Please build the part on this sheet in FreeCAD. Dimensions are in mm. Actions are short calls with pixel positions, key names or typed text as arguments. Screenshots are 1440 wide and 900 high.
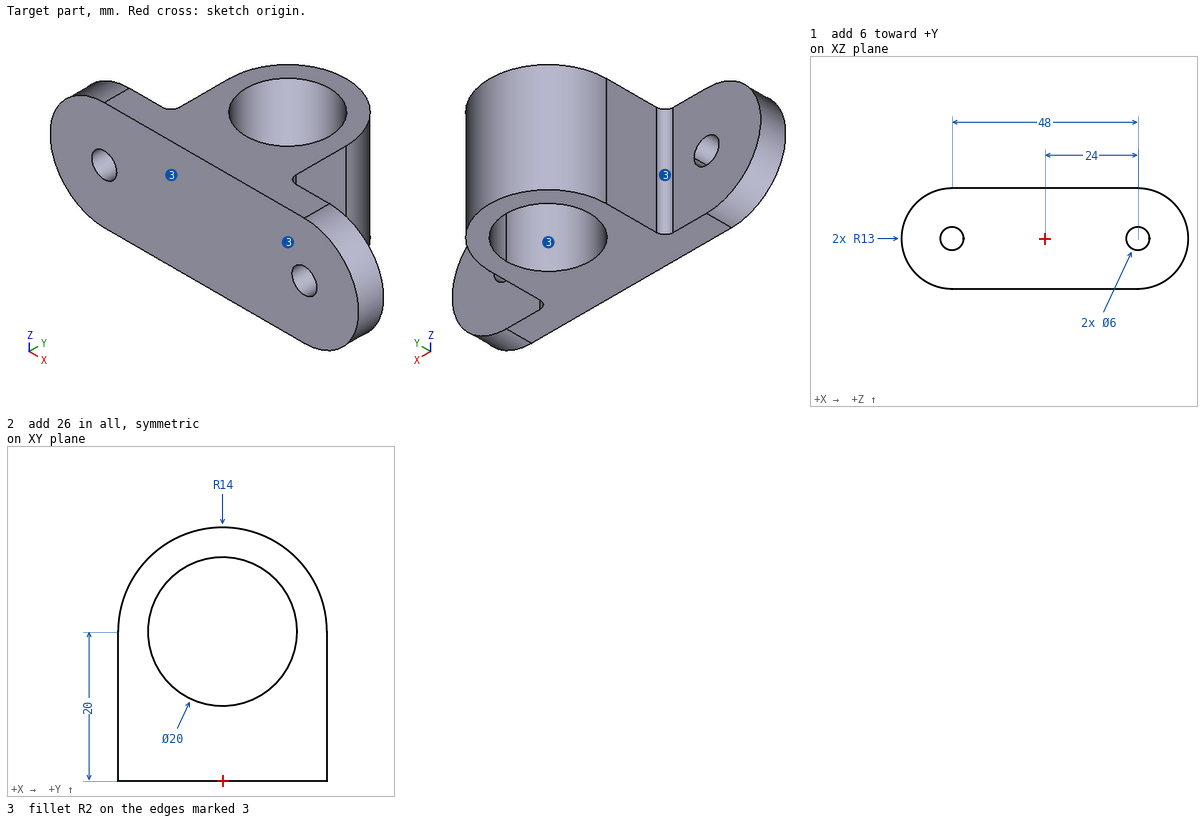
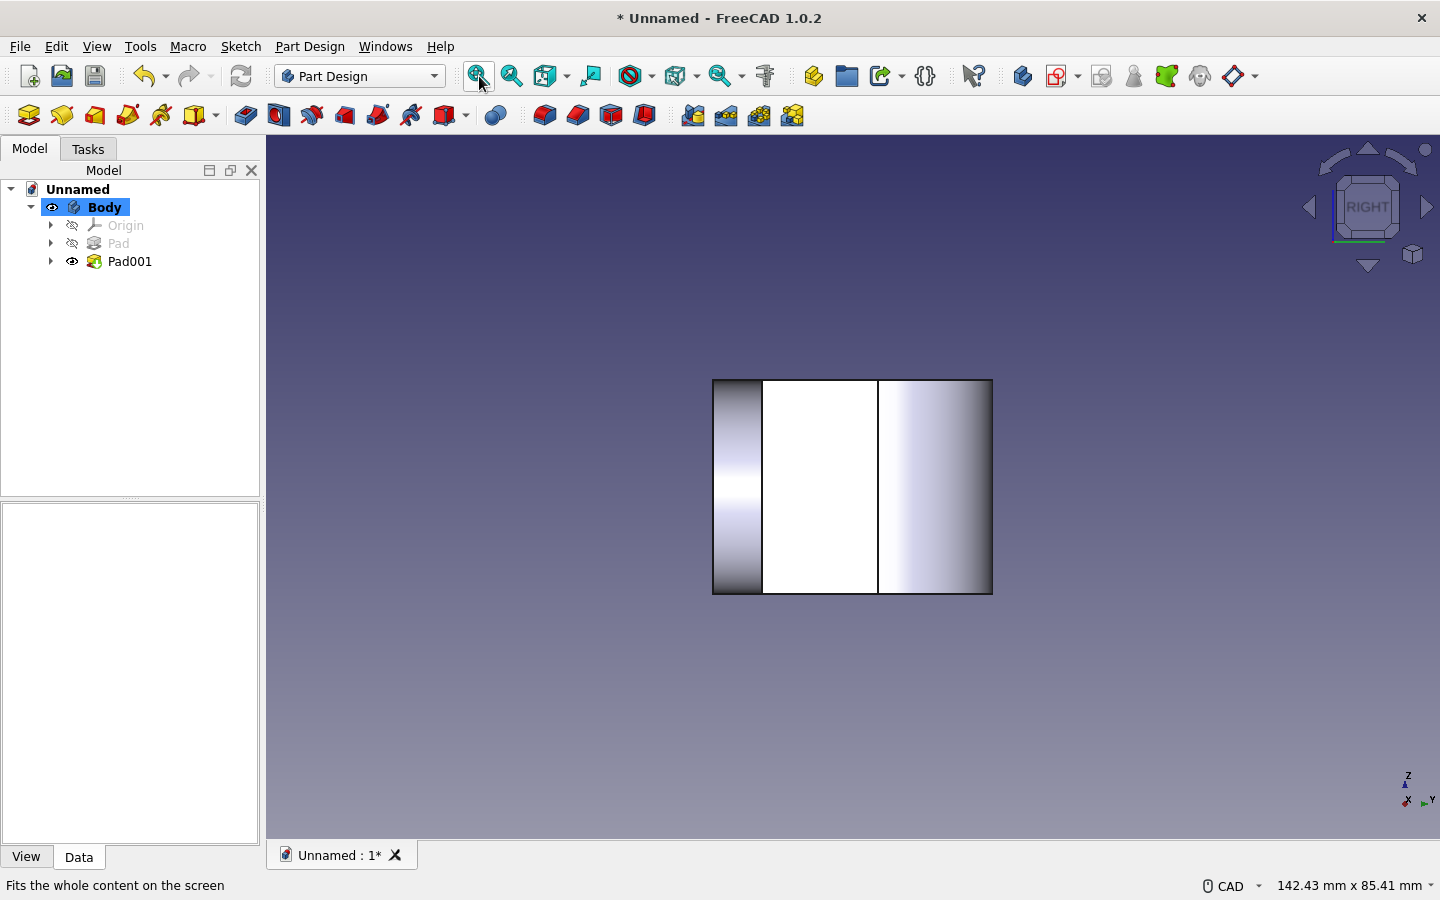
key(5)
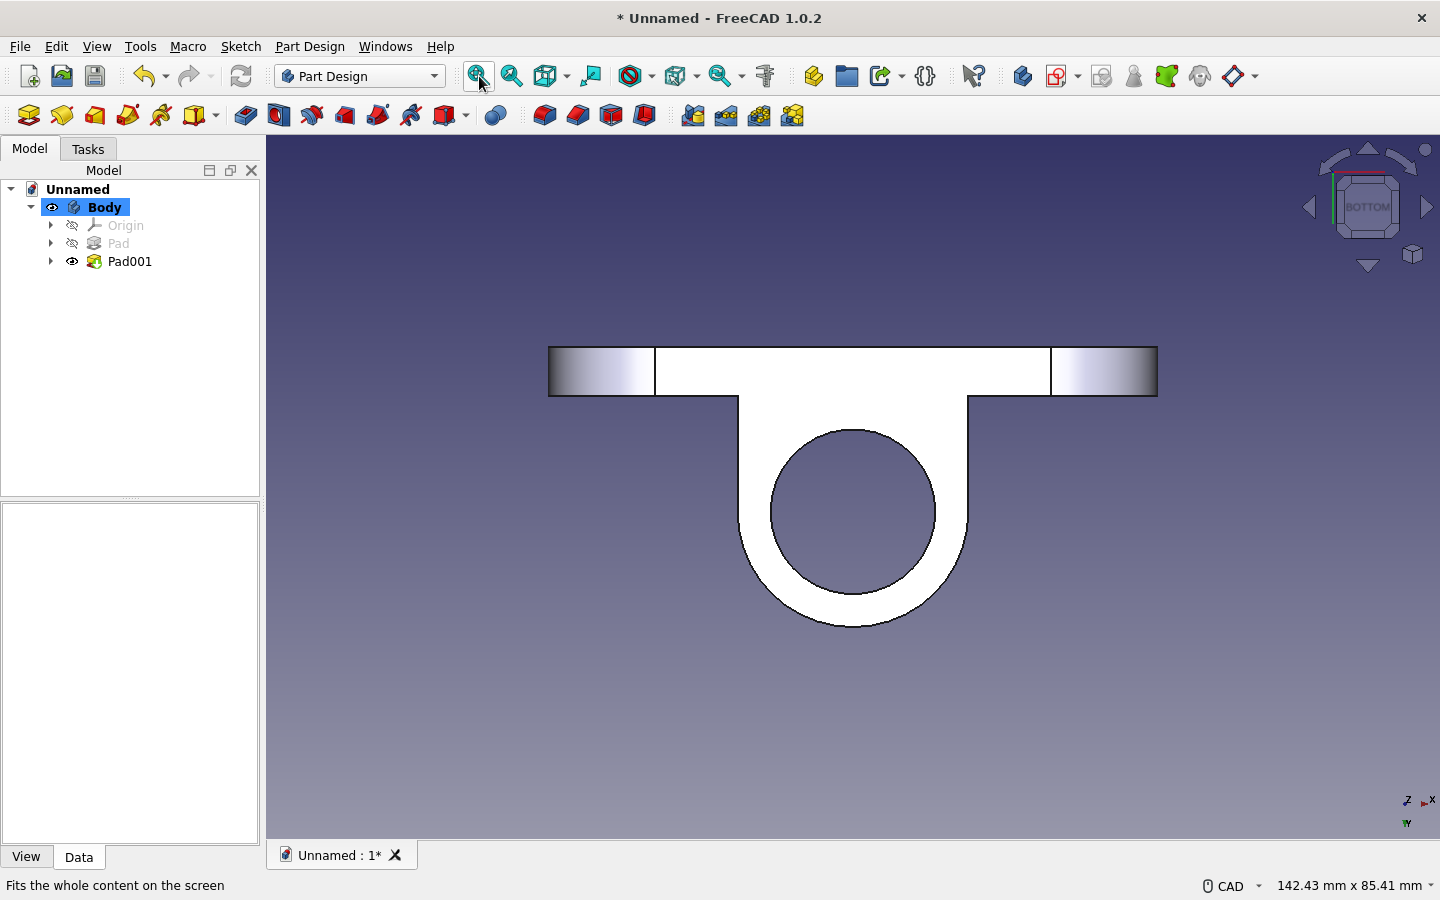
key(4)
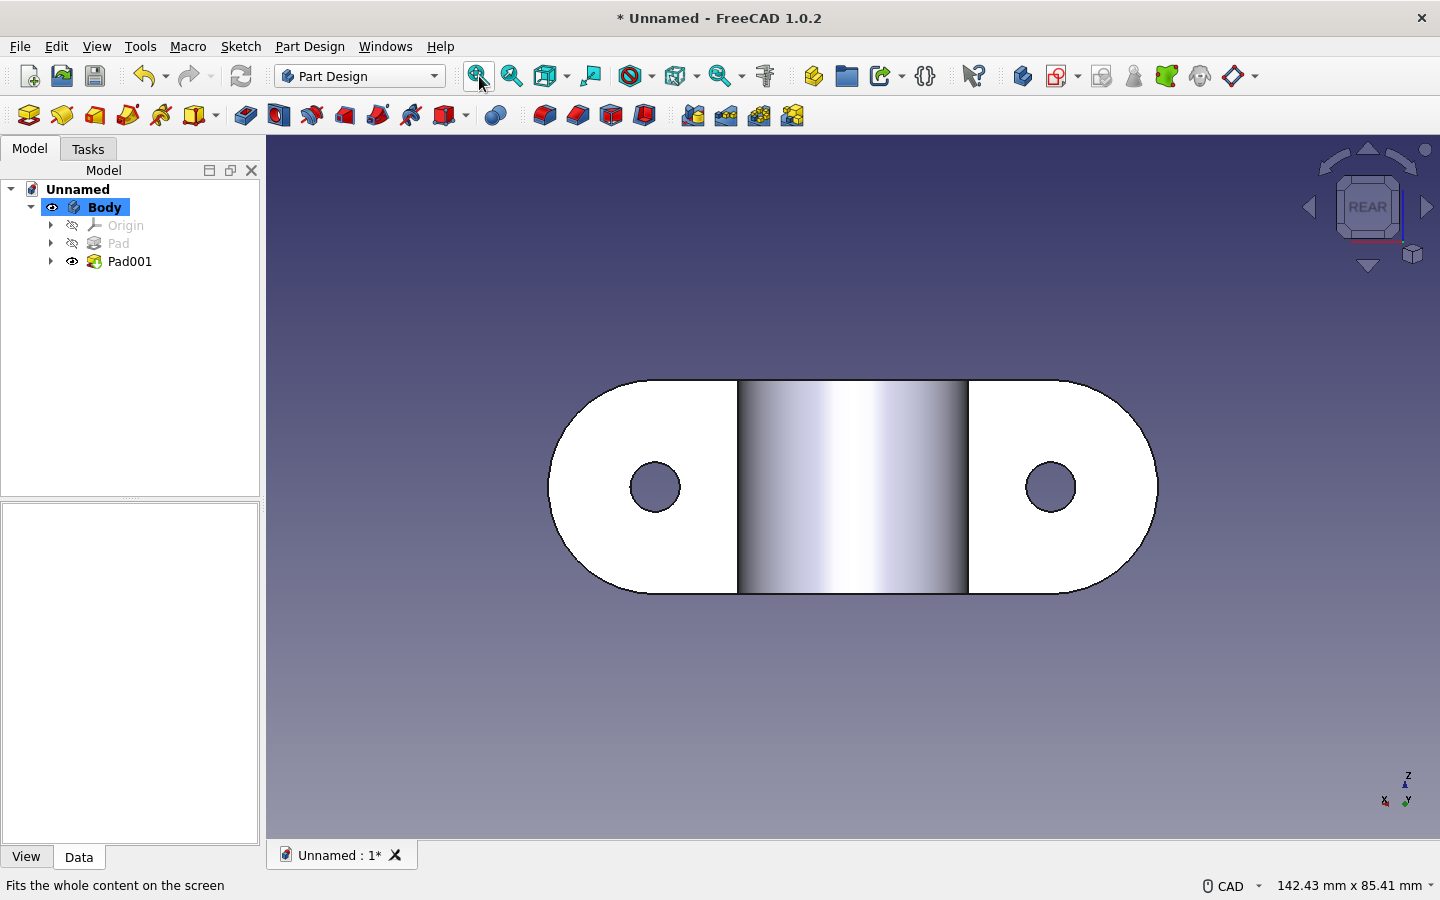
key(6)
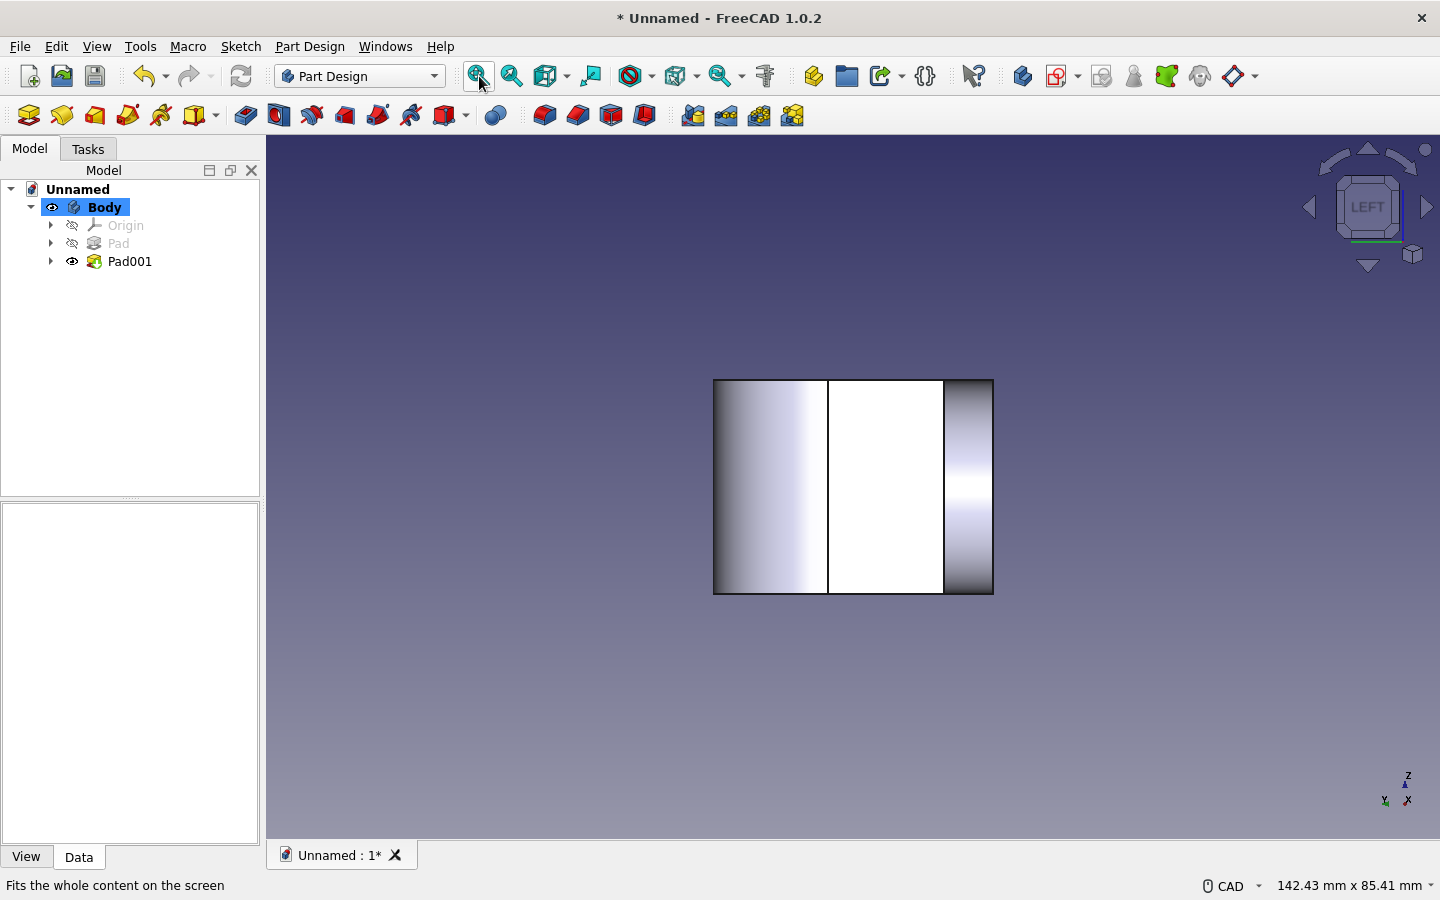
key(v)
key(f)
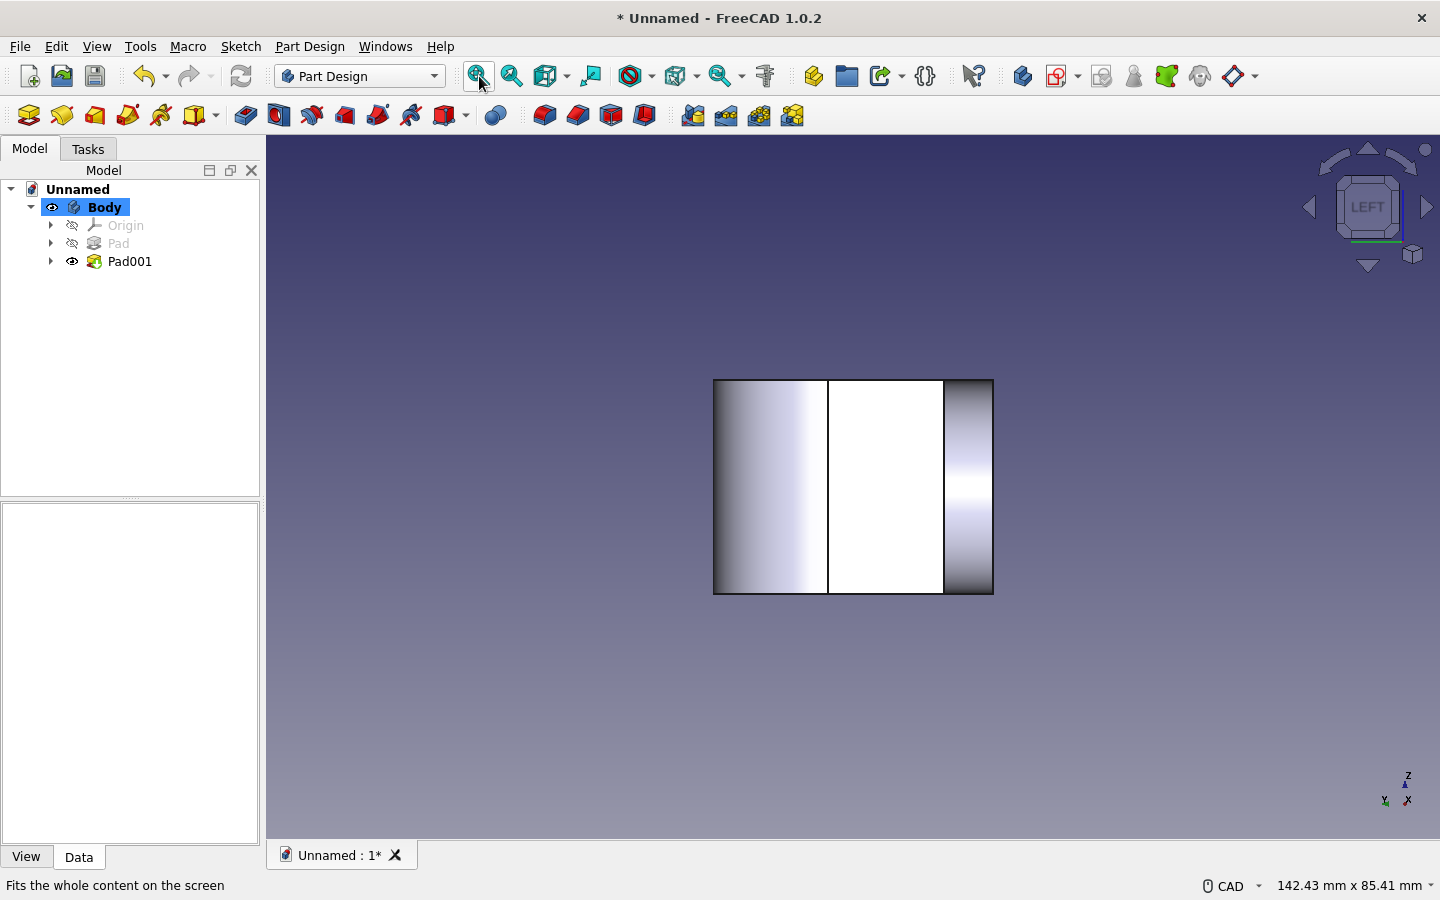
key(v)
key(3)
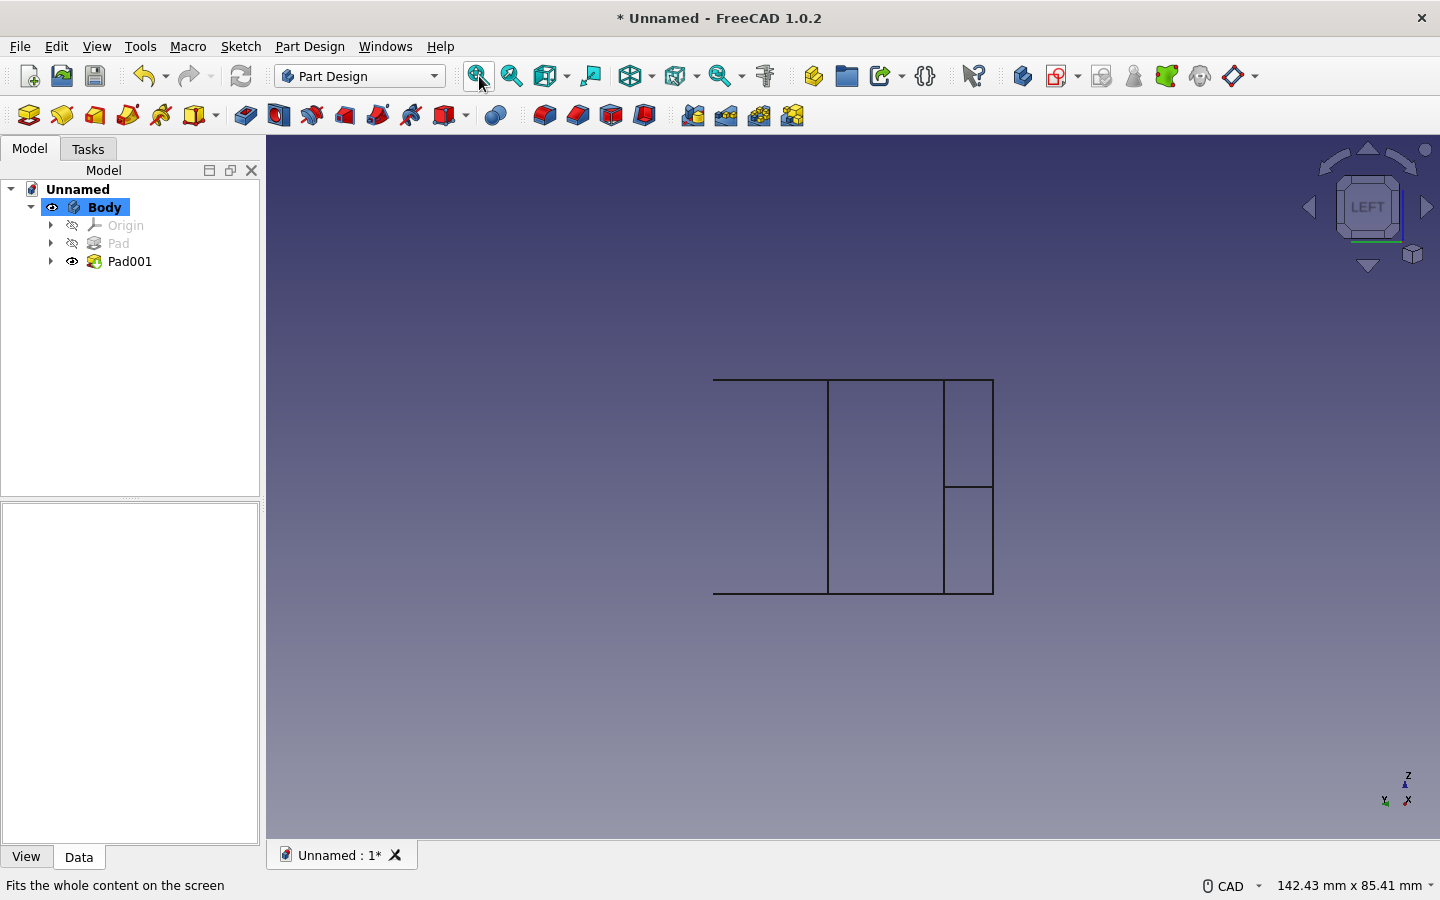
key(0)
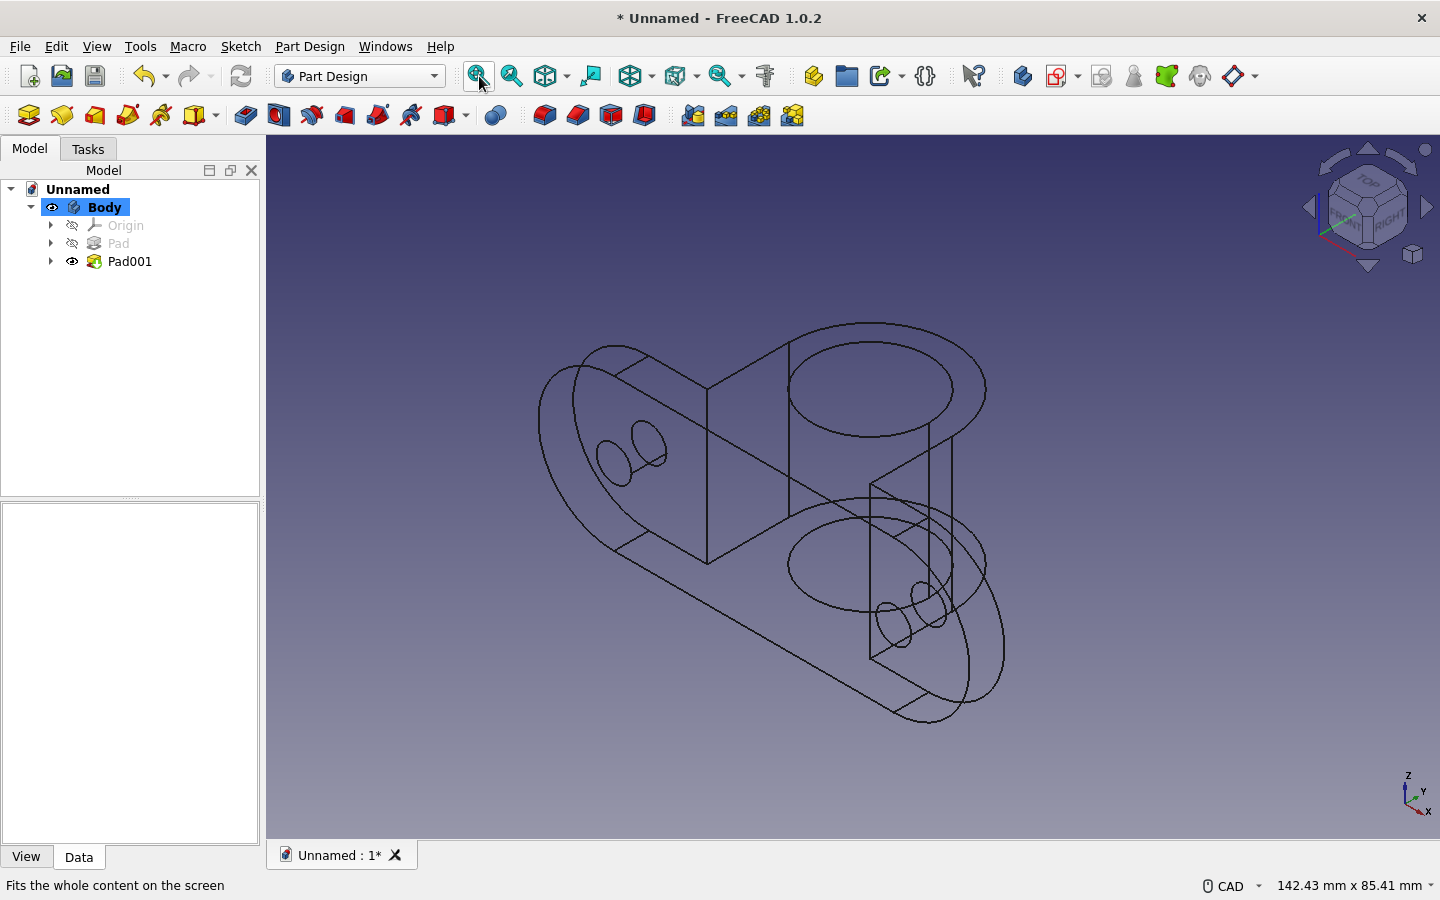
click(707, 476)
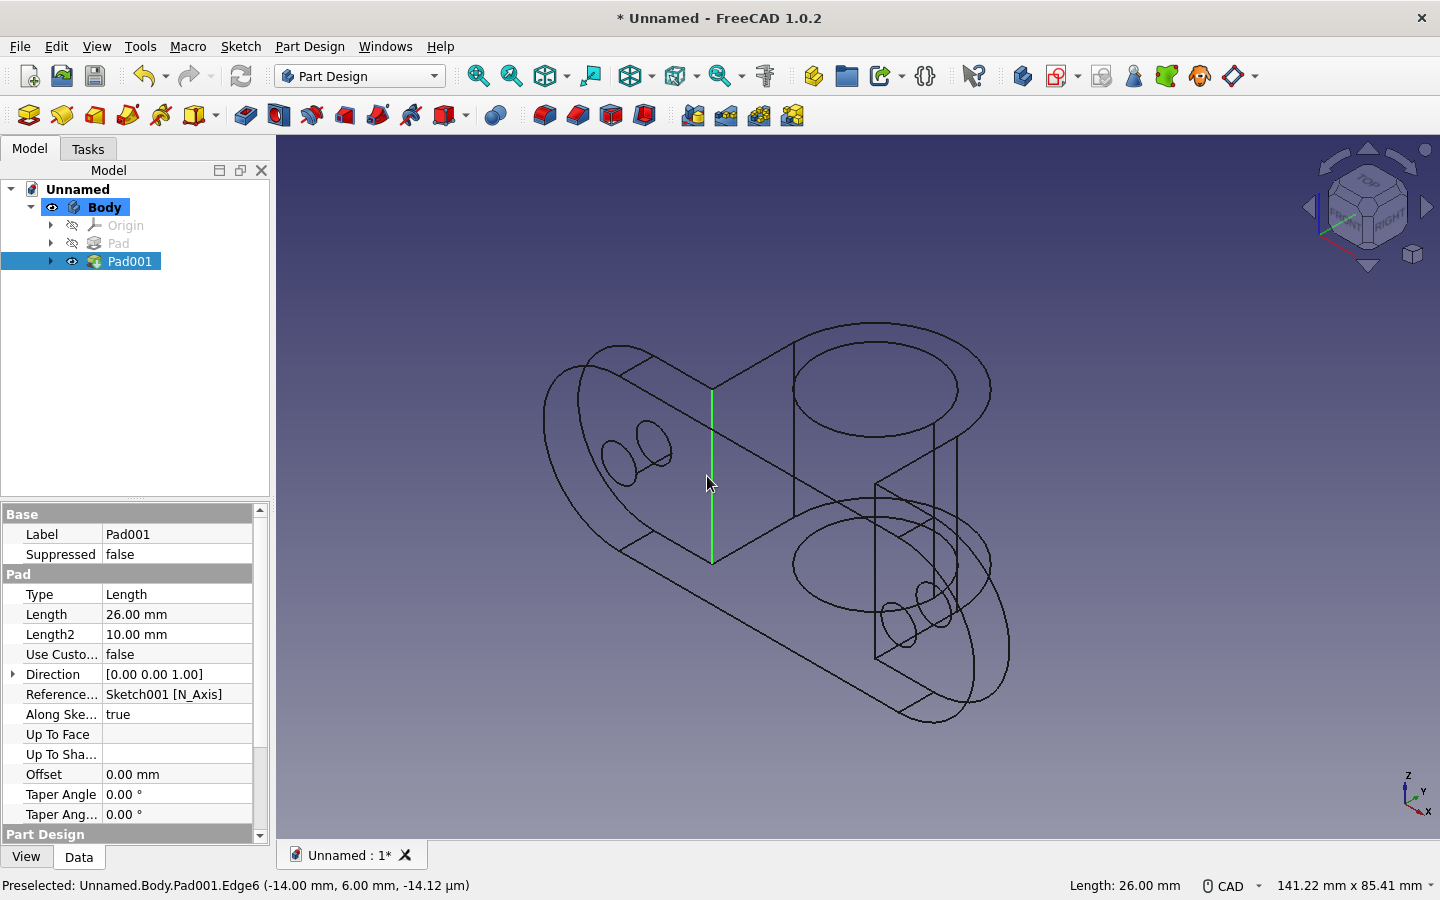
click(875, 570, ctrl)